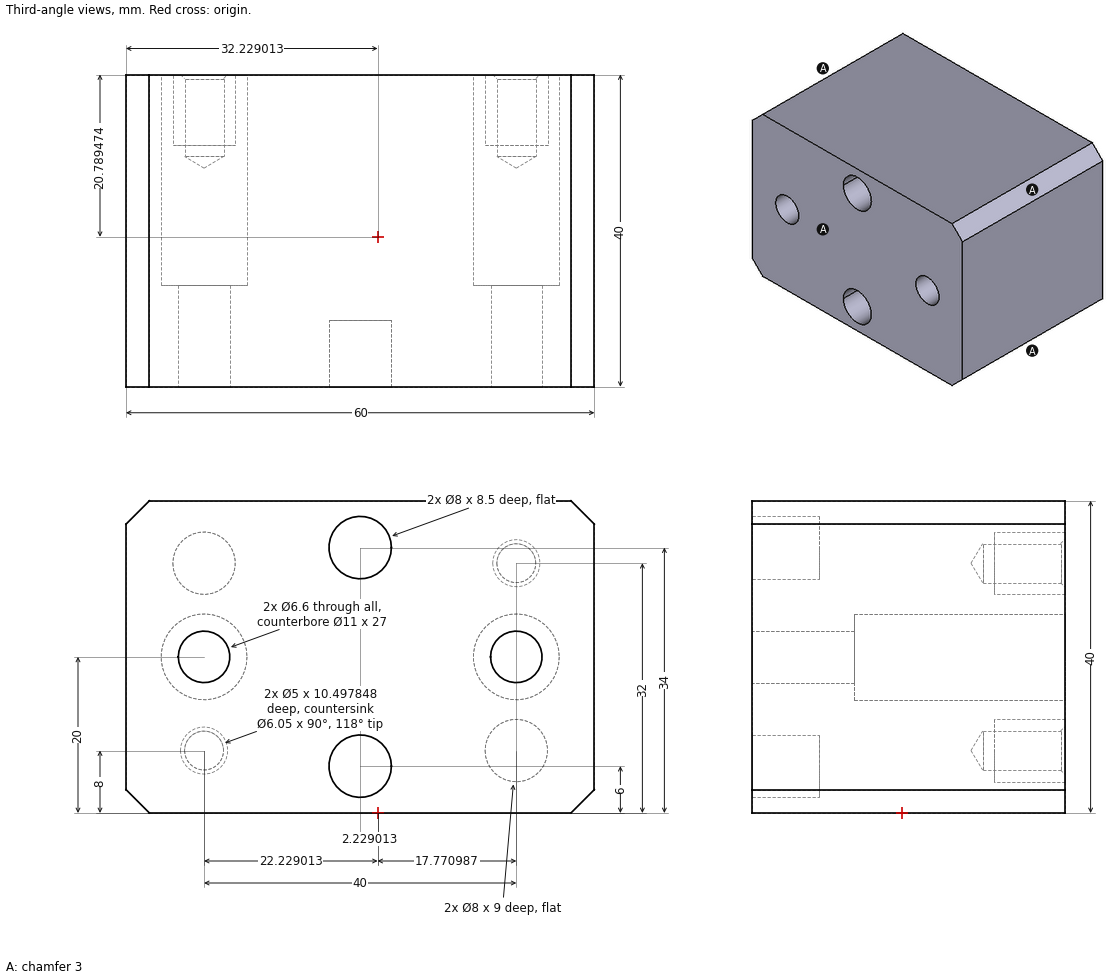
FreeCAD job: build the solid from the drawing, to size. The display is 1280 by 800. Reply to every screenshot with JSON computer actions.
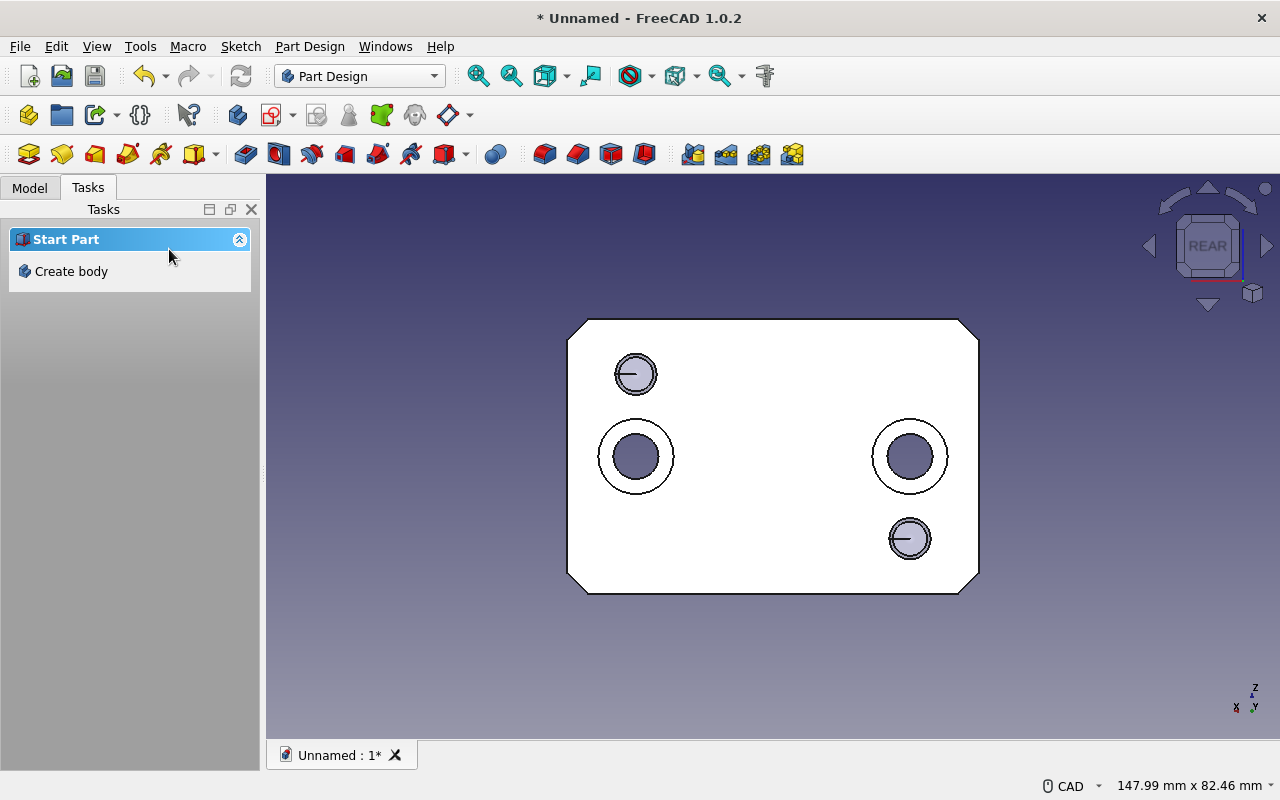
{"action": "left_click", "coordinate": [773, 455]}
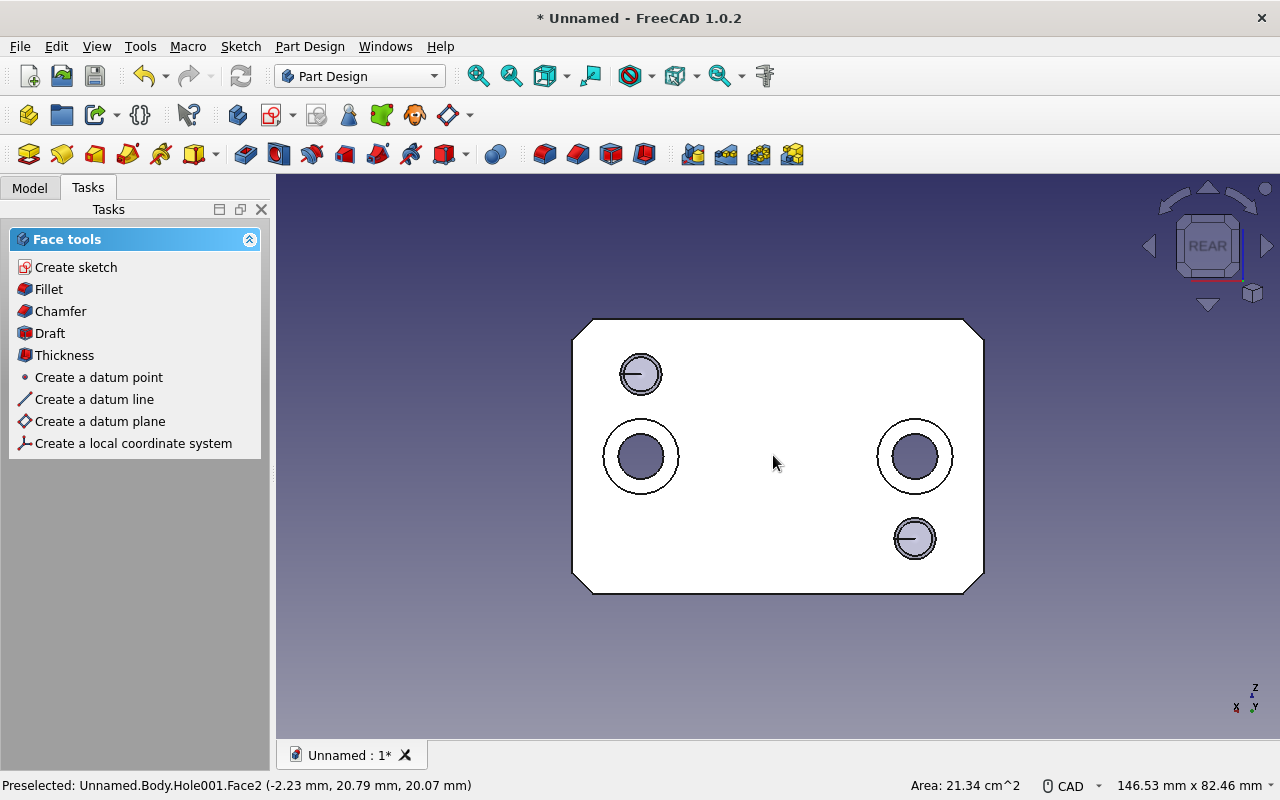
{"action": "left_click", "coordinate": [270, 116]}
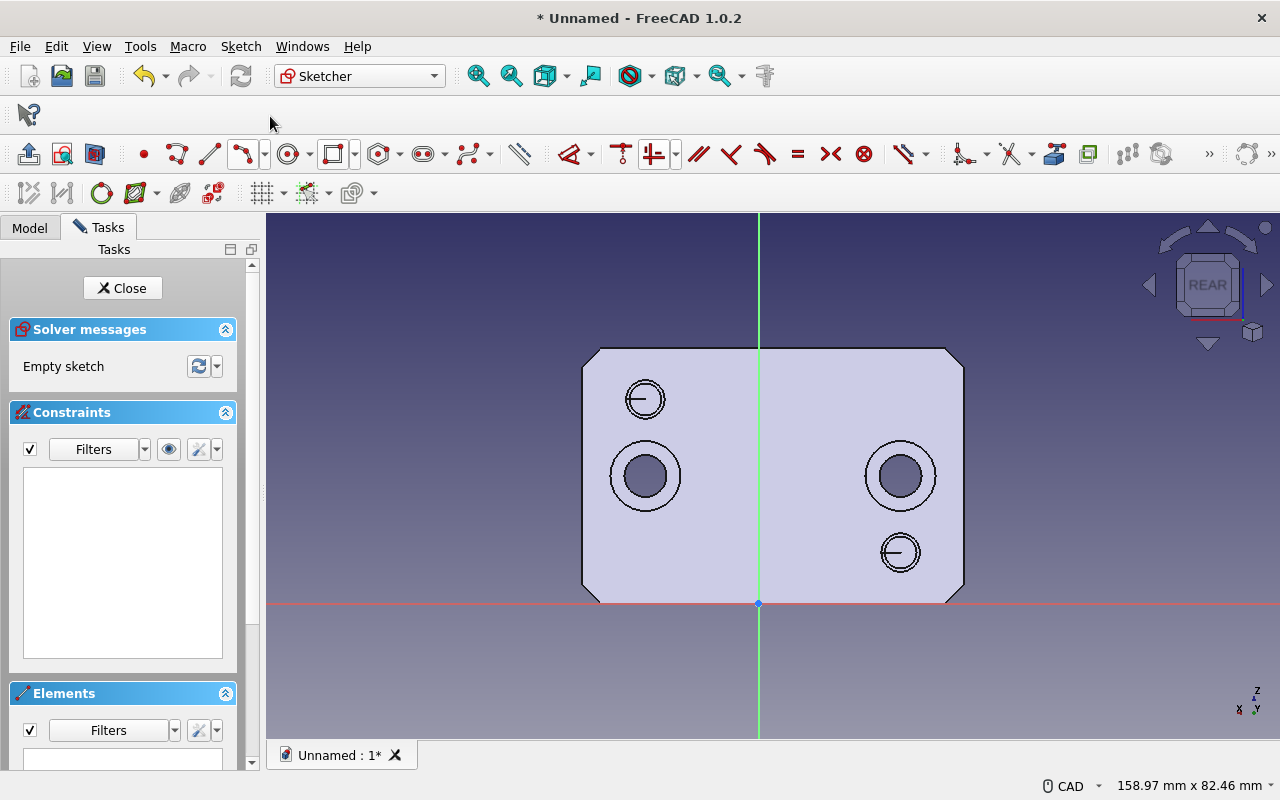
{"action": "scroll", "coordinate": [912, 515], "scroll_direction": "up", "scroll_amount": 2}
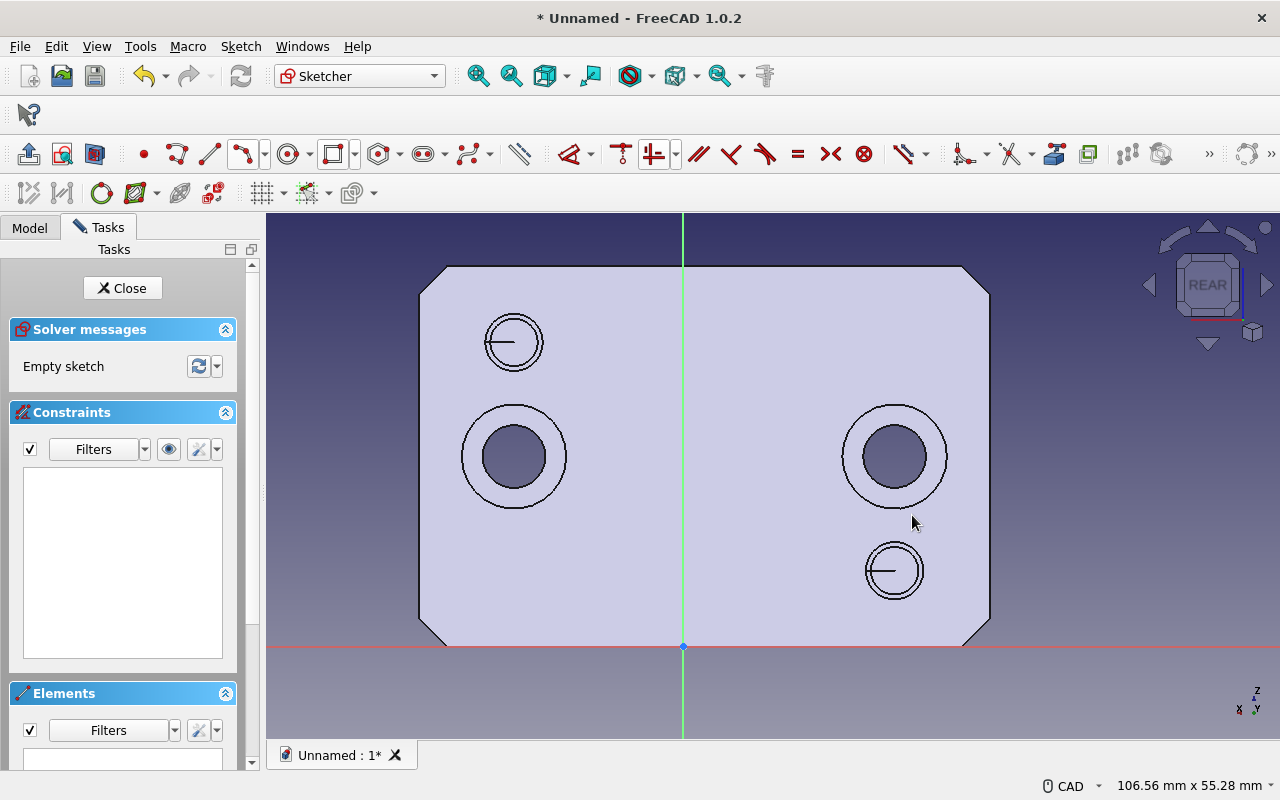
{"action": "key", "text": "g c"}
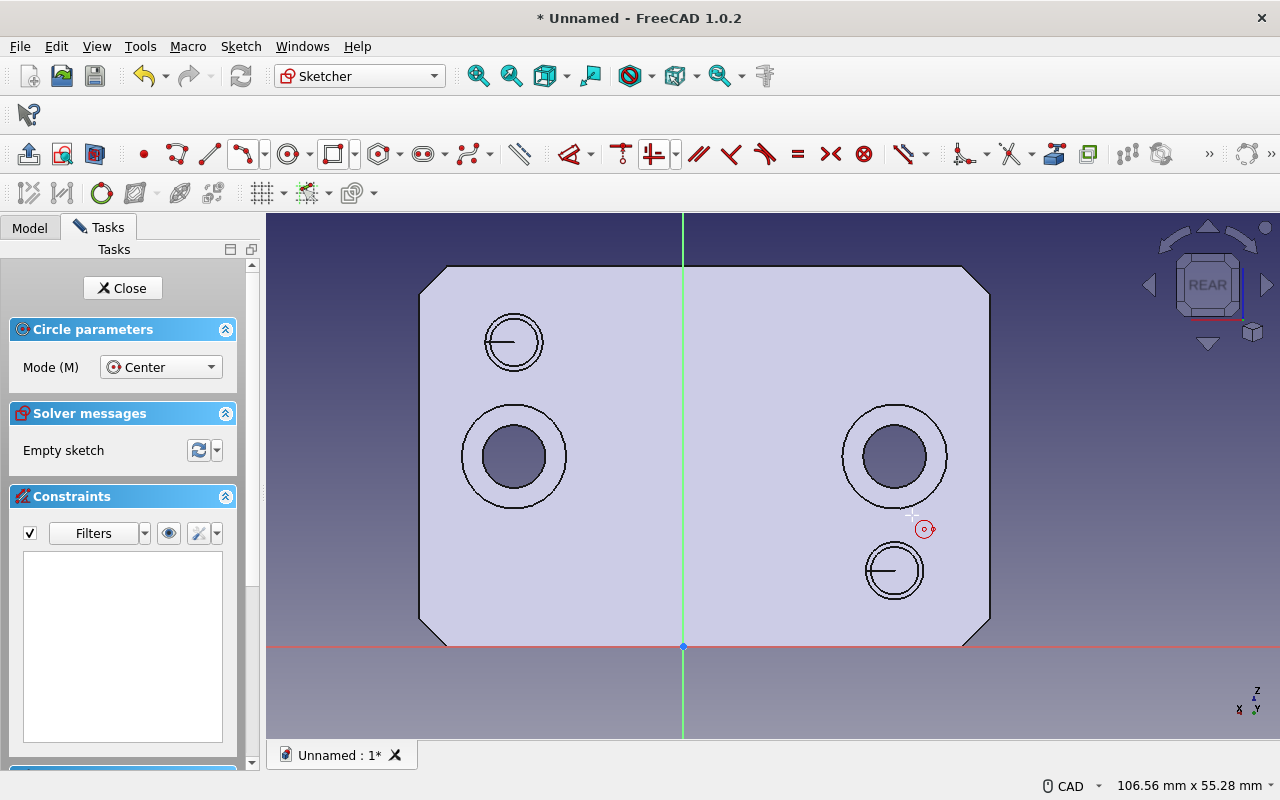
{"action": "left_click", "coordinate": [514, 571]}
{"action": "mouse_move", "coordinate": [541, 544]}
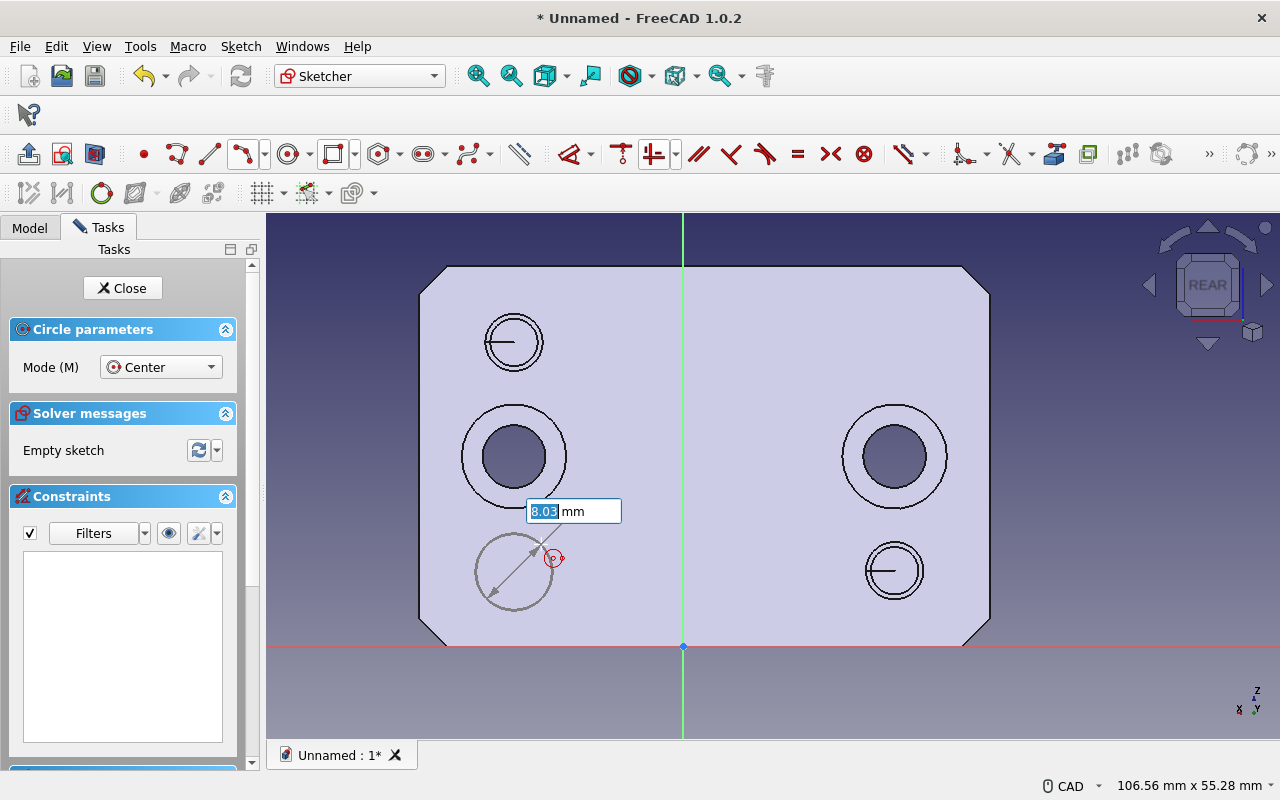
{"action": "type", "text": "8"}
{"action": "key", "text": "Return"}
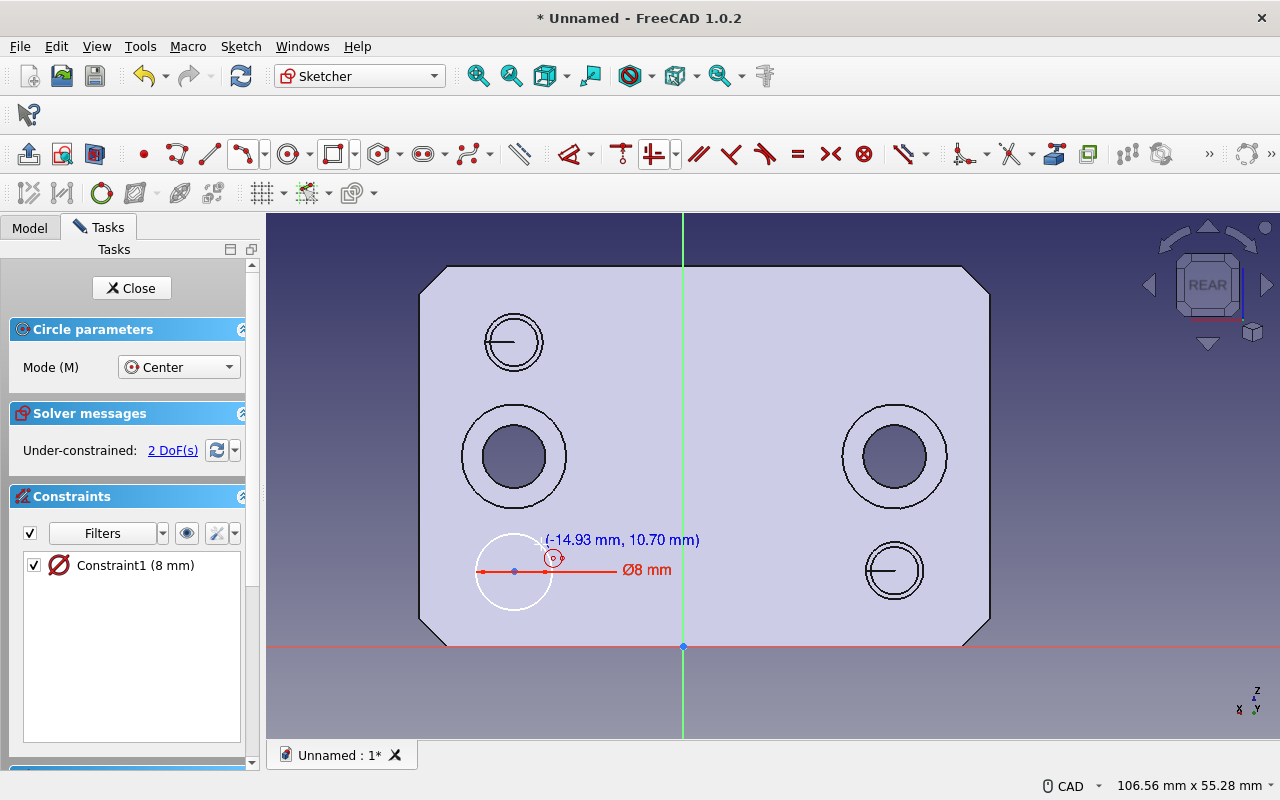
{"action": "left_click", "coordinate": [895, 342]}
{"action": "mouse_move", "coordinate": [922, 315]}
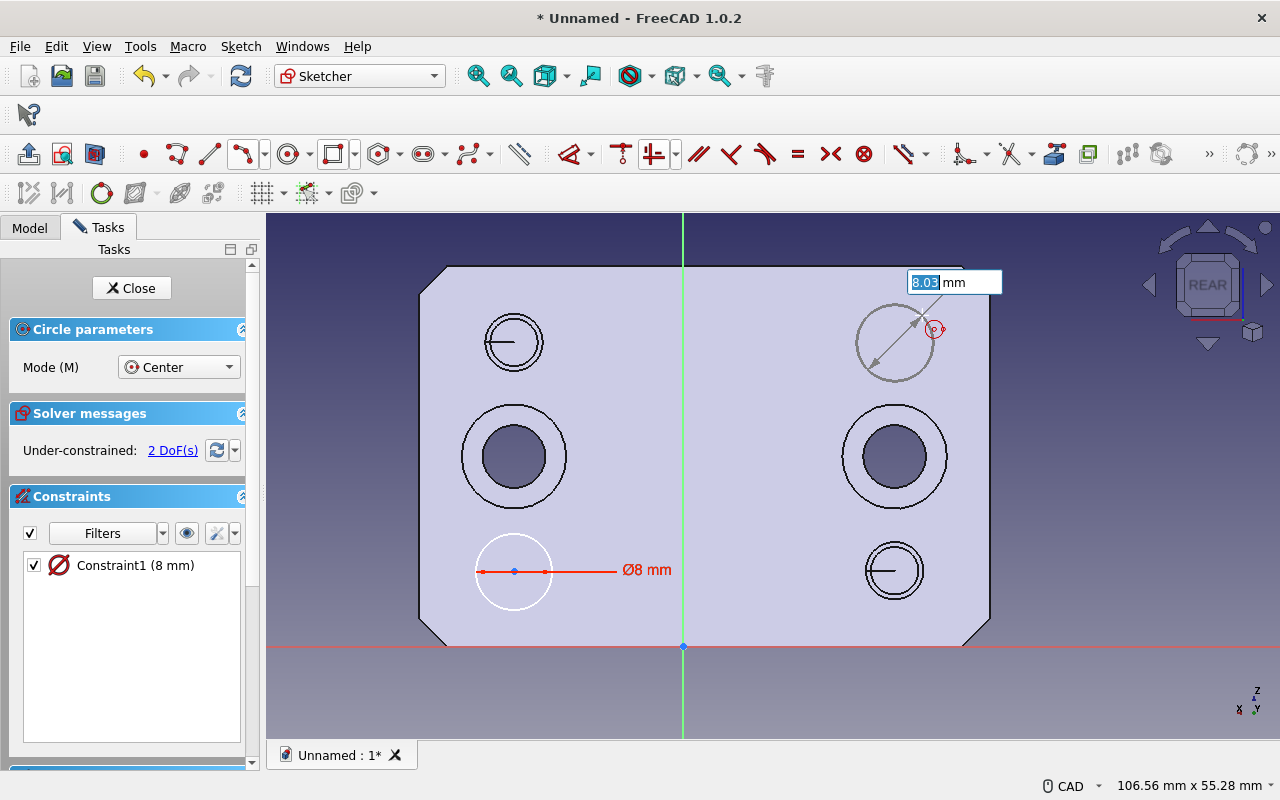
{"action": "type", "text": "8"}
{"action": "key", "text": "Return"}
{"action": "key", "text": "Escape"}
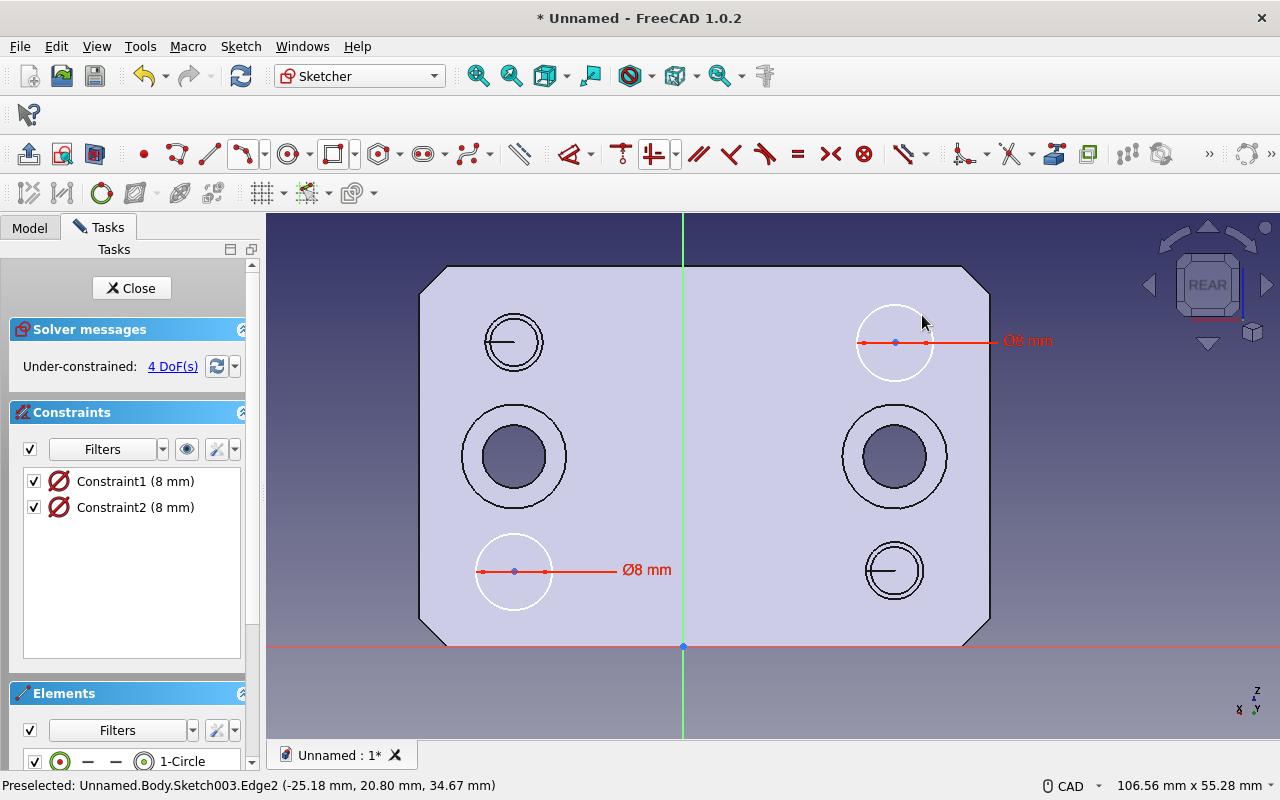
{"action": "key", "text": "d"}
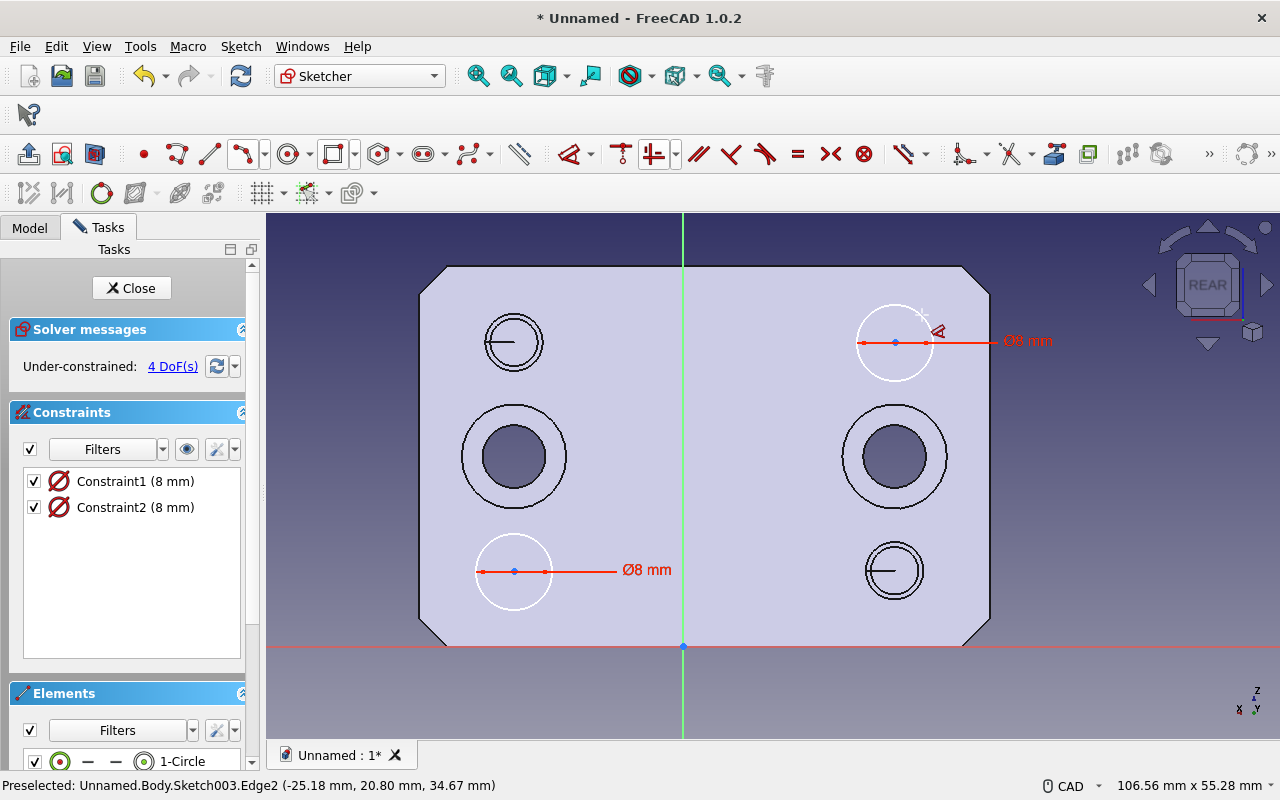
{"action": "left_click", "coordinate": [514, 572]}
{"action": "left_click", "coordinate": [480, 627]}